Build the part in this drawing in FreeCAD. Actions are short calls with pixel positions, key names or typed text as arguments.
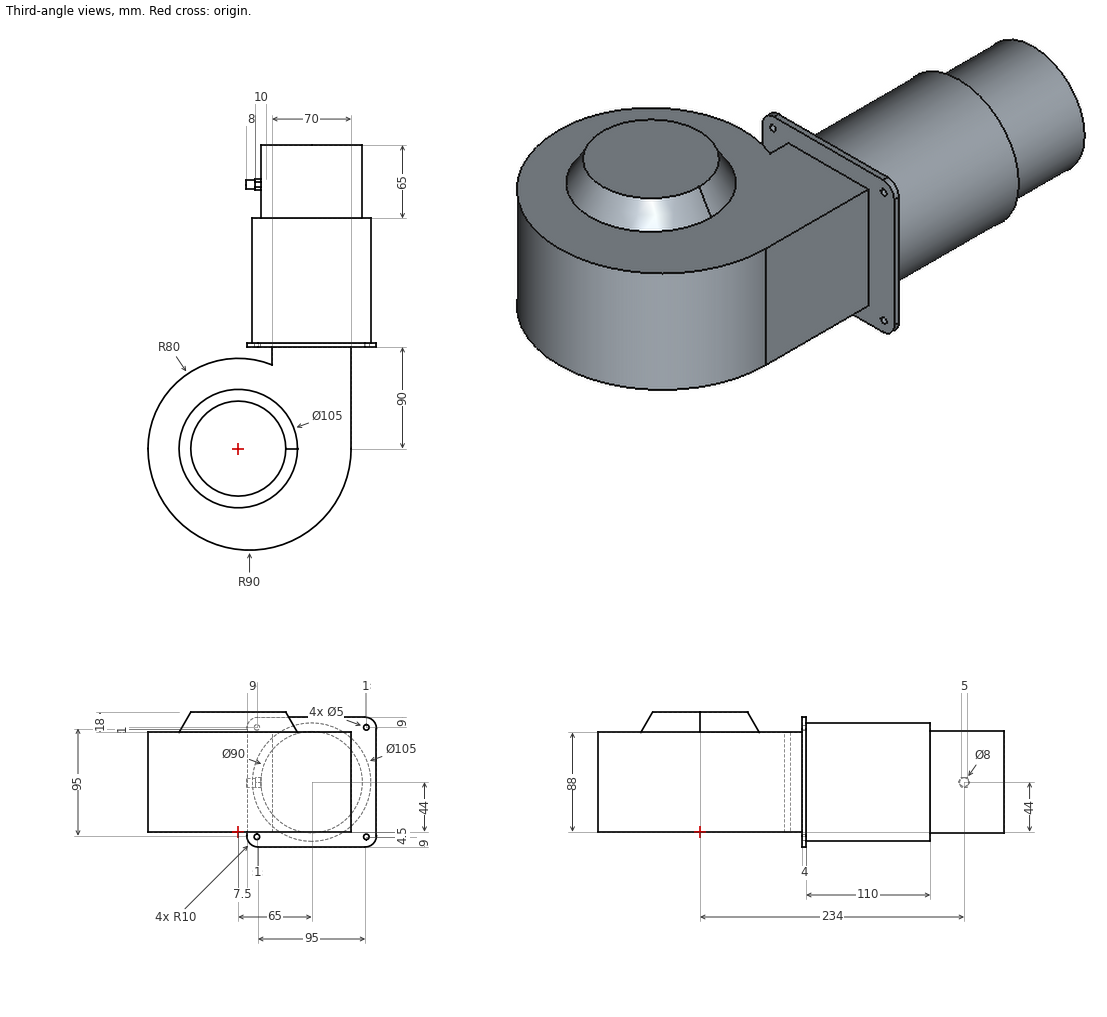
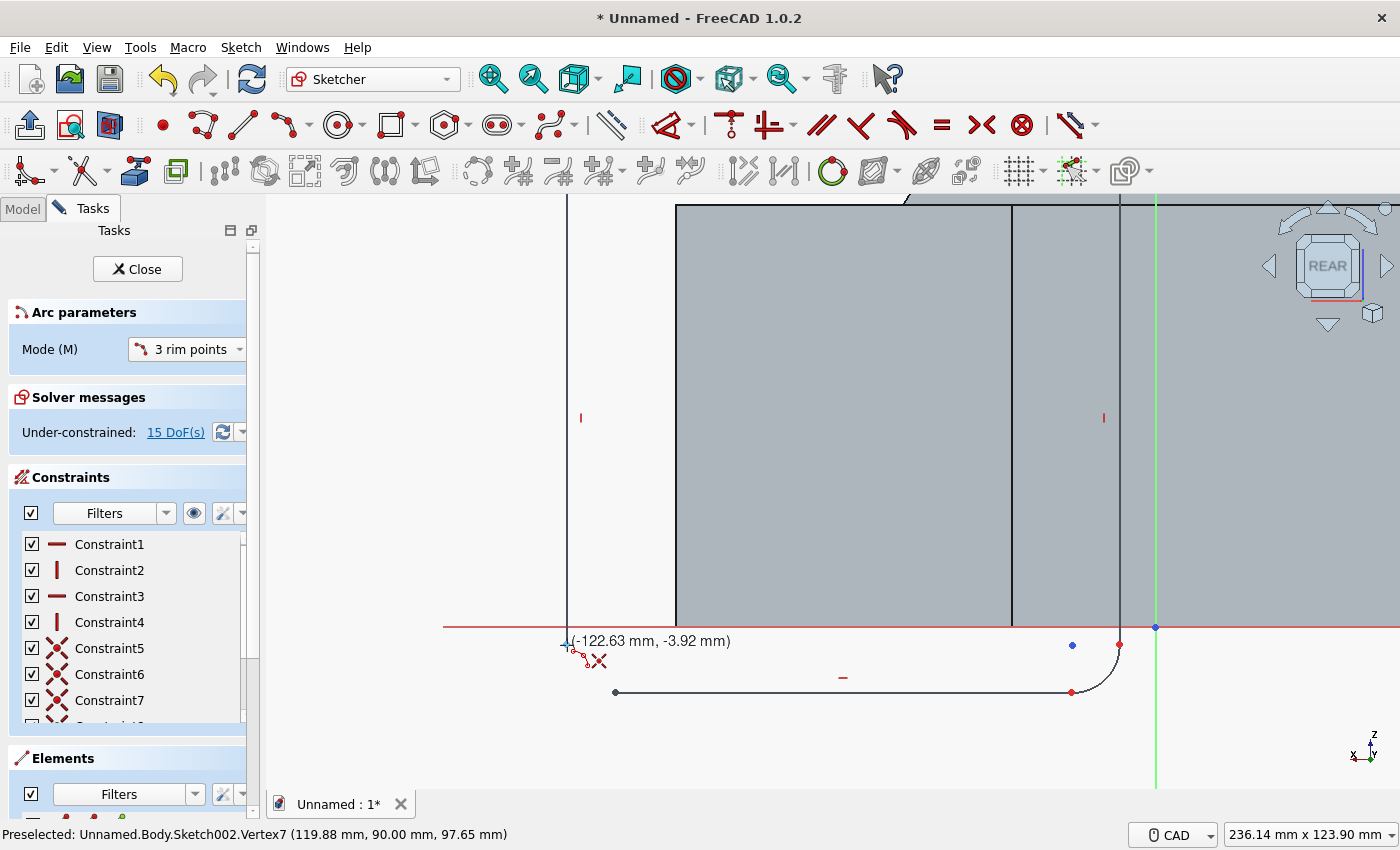
click(567, 645)
click(615, 693)
click(582, 678)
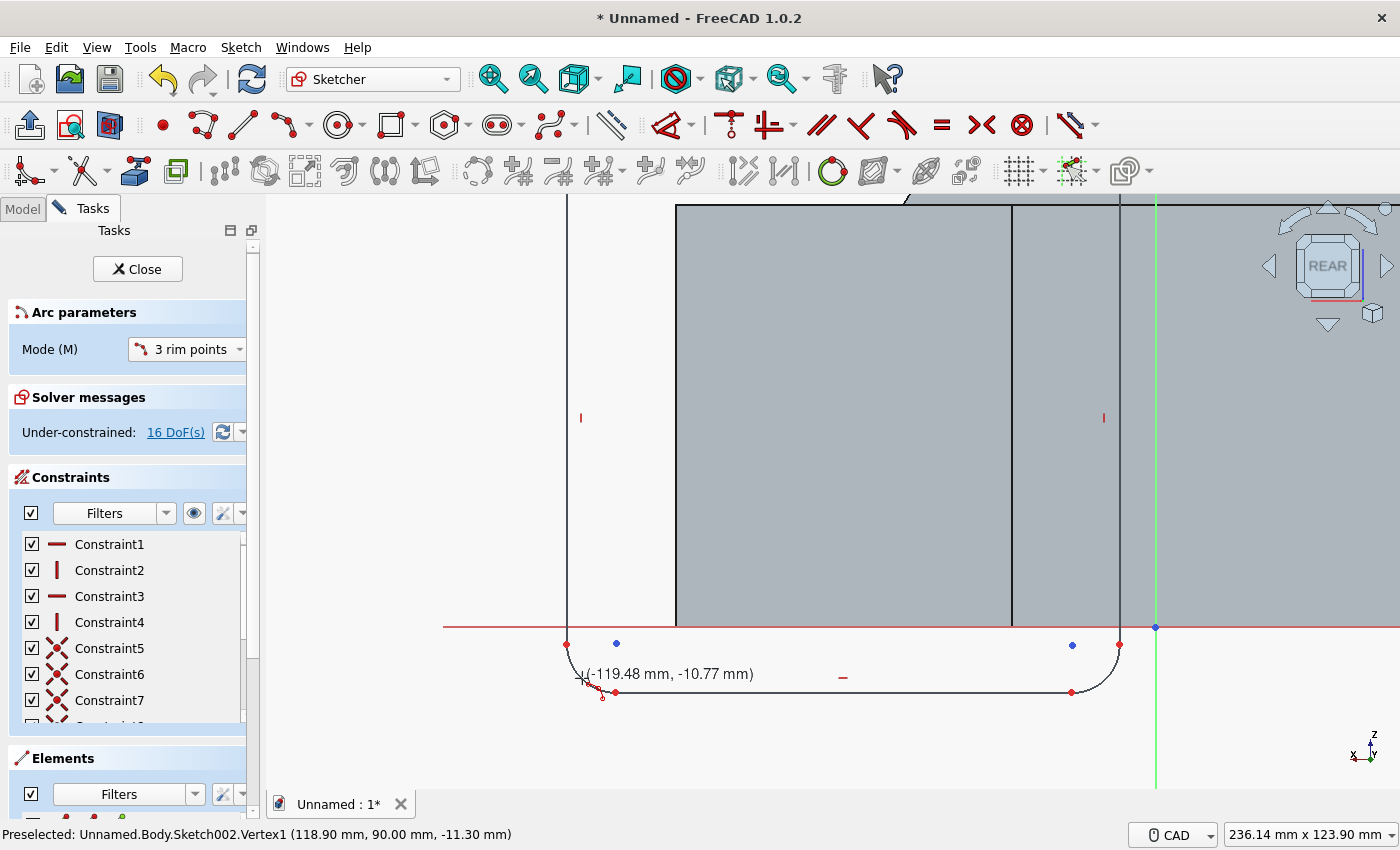
click(338, 126)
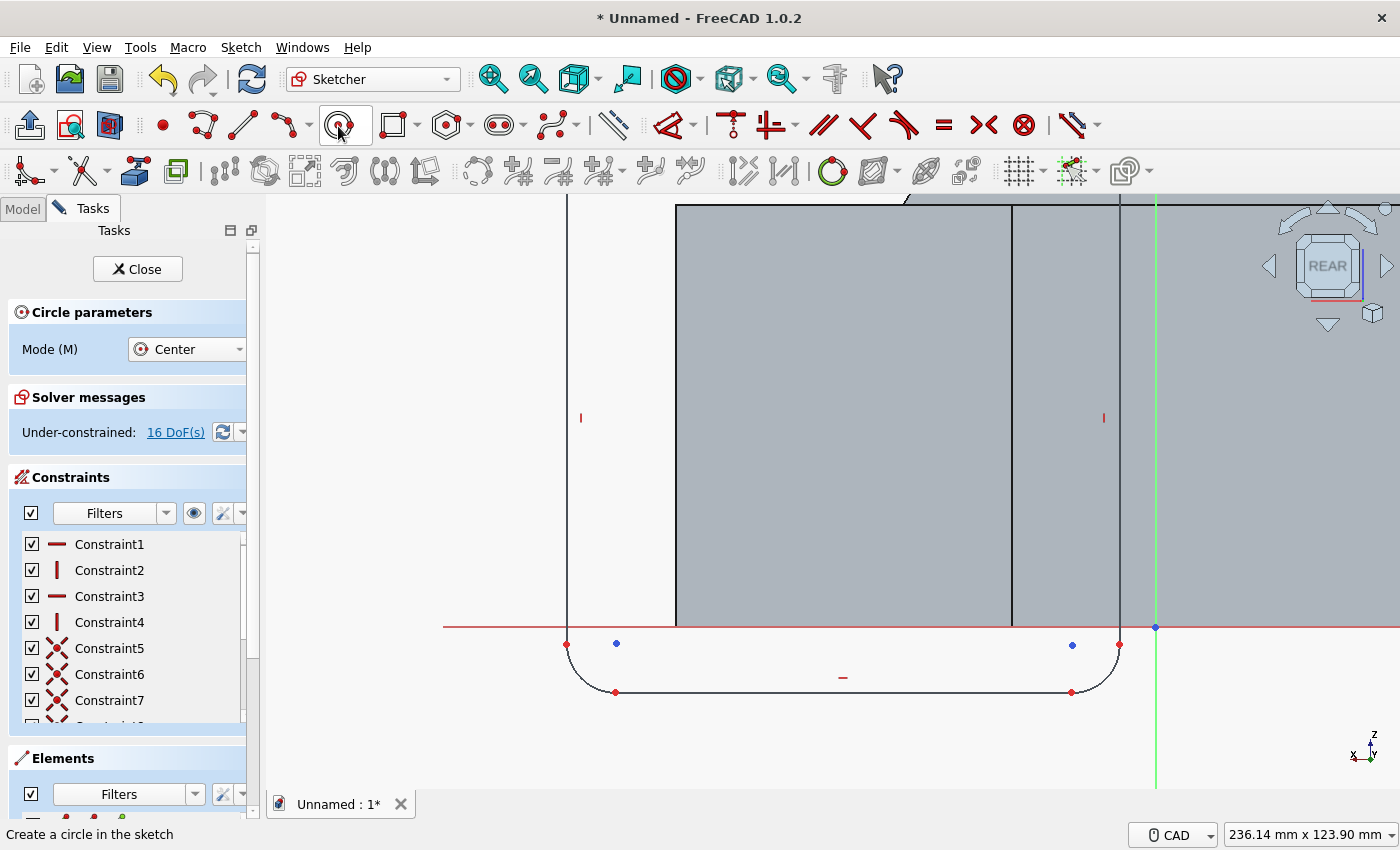
scroll(567, 645, down, 2)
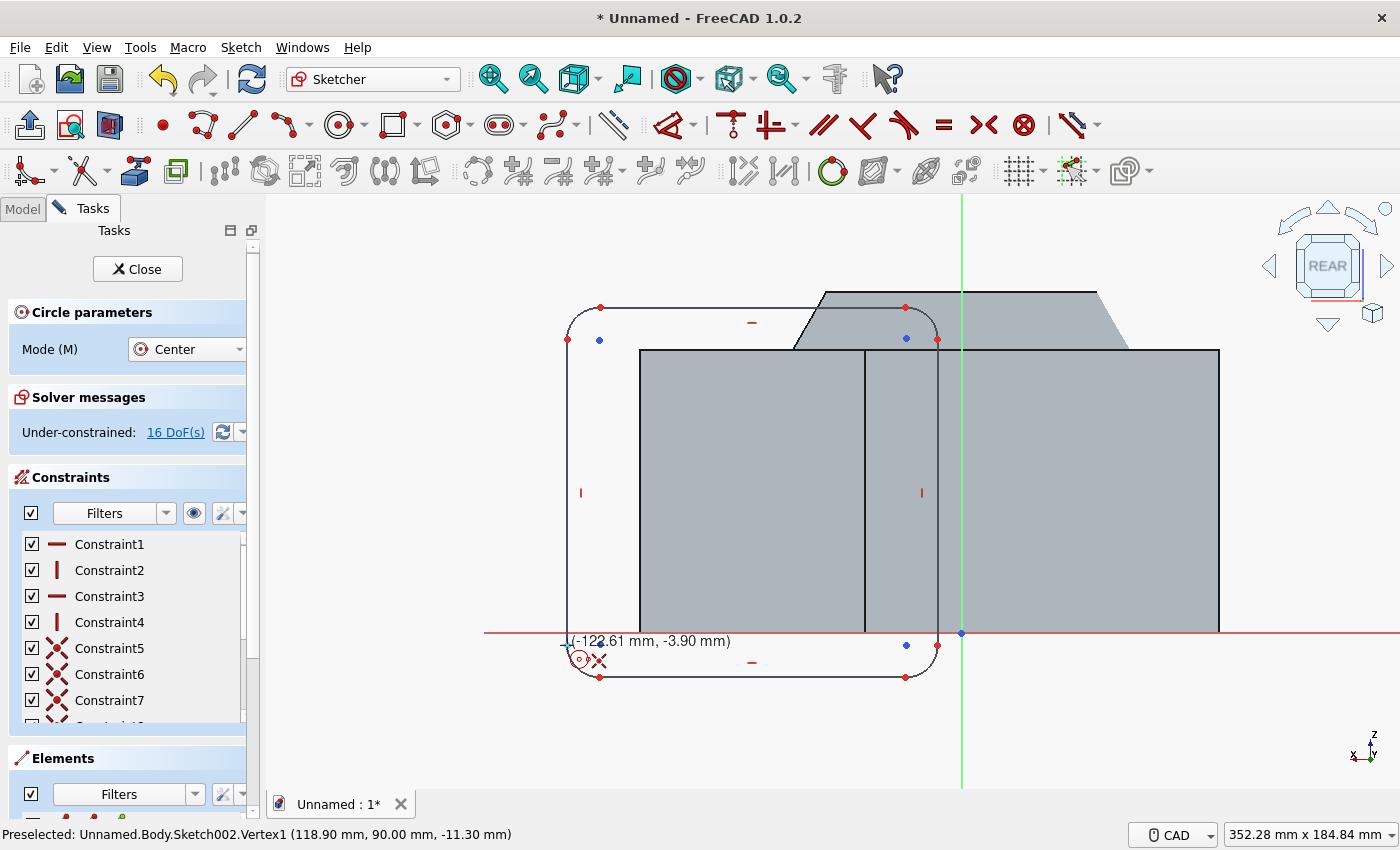
scroll(596, 336, up, 7)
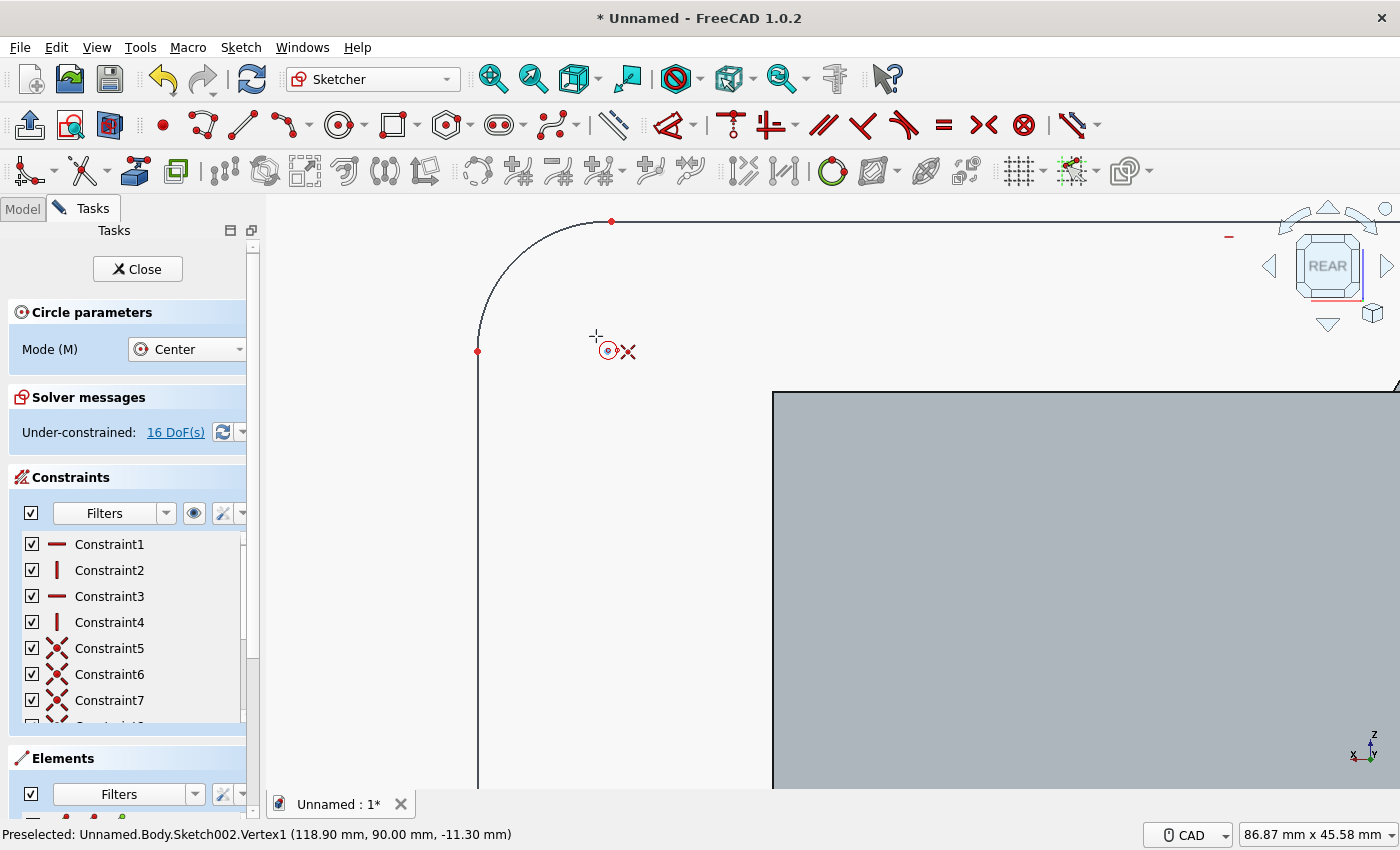
click(597, 334)
click(620, 311)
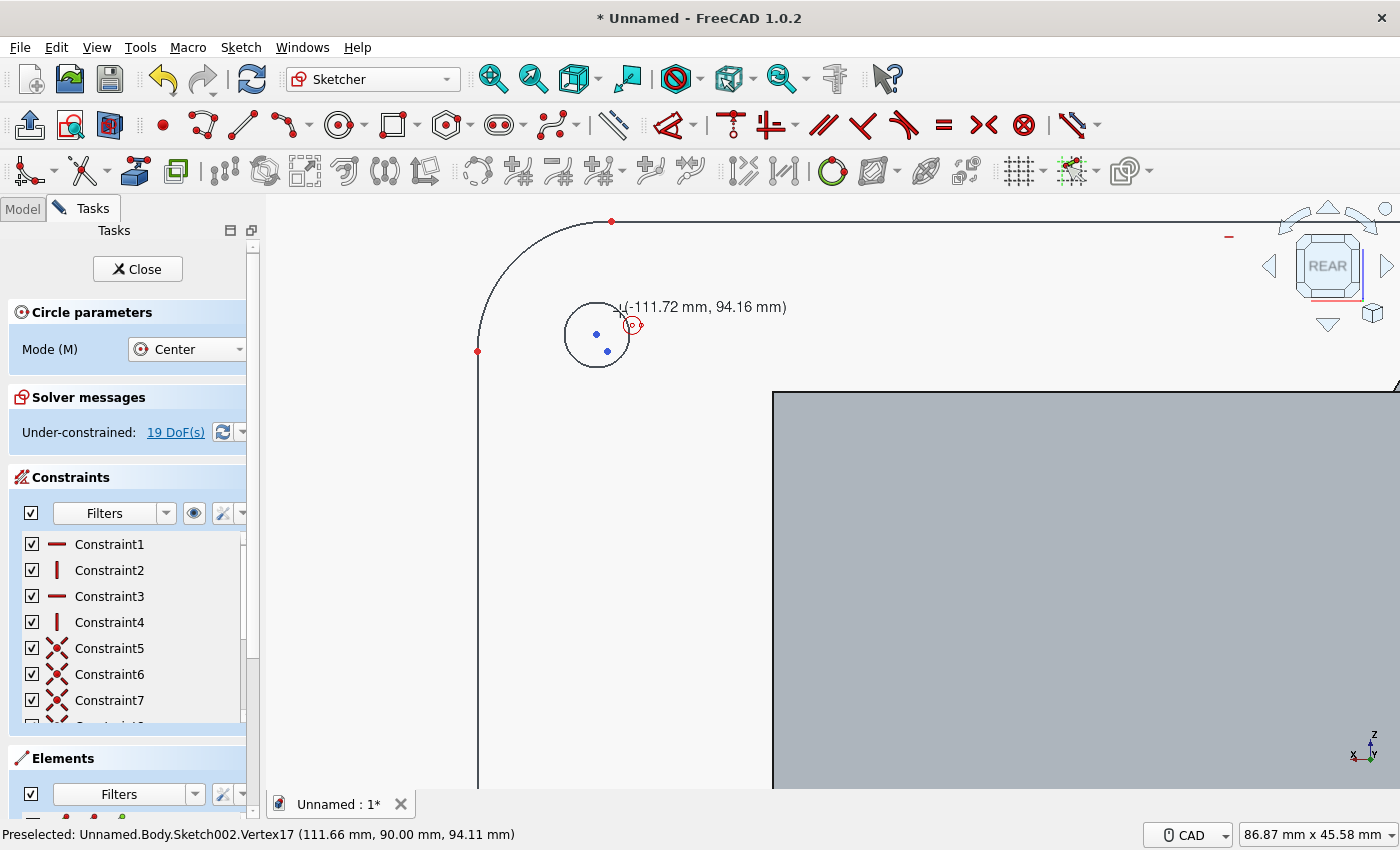
scroll(596, 336, down, 7)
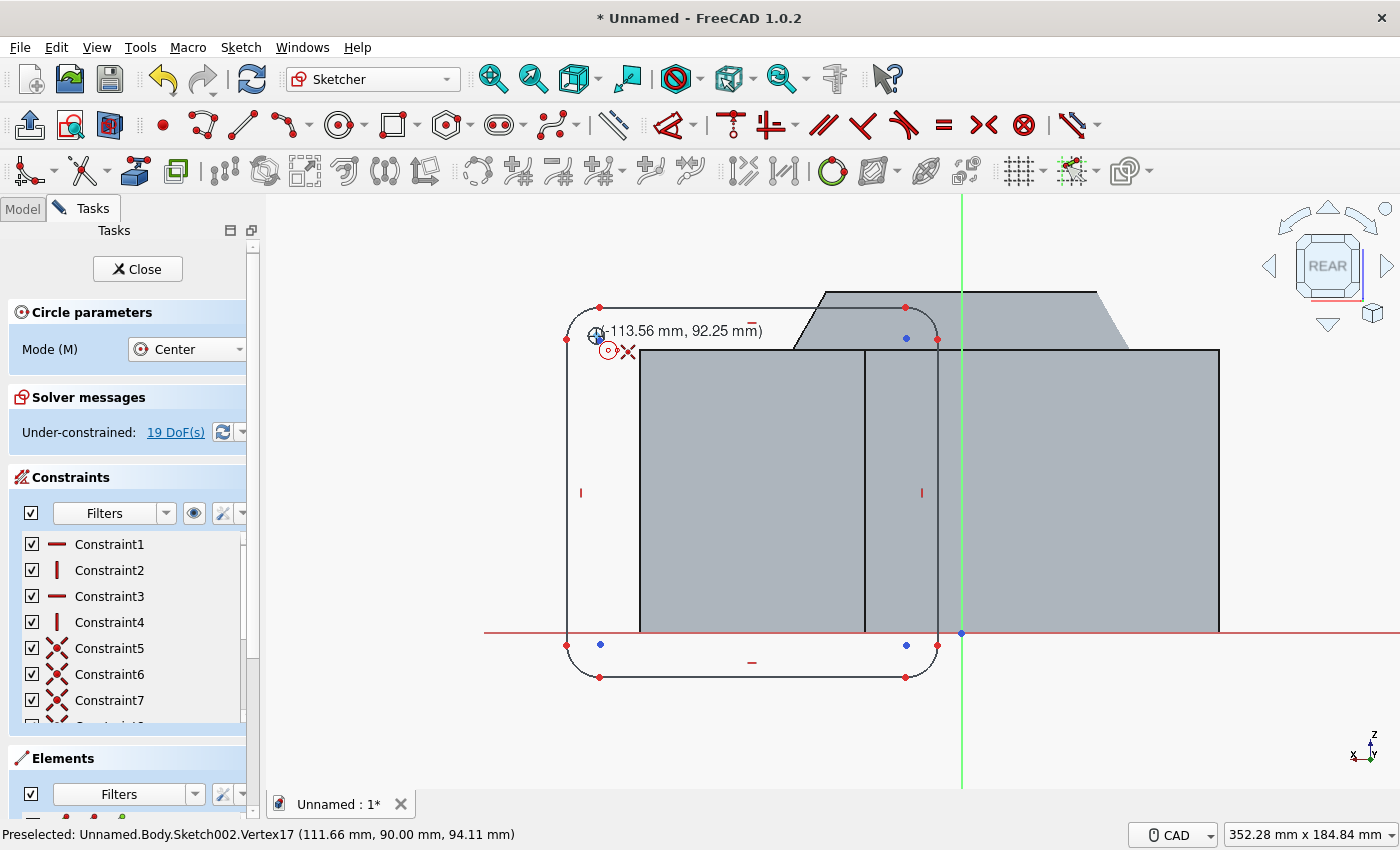
scroll(909, 336, up, 7)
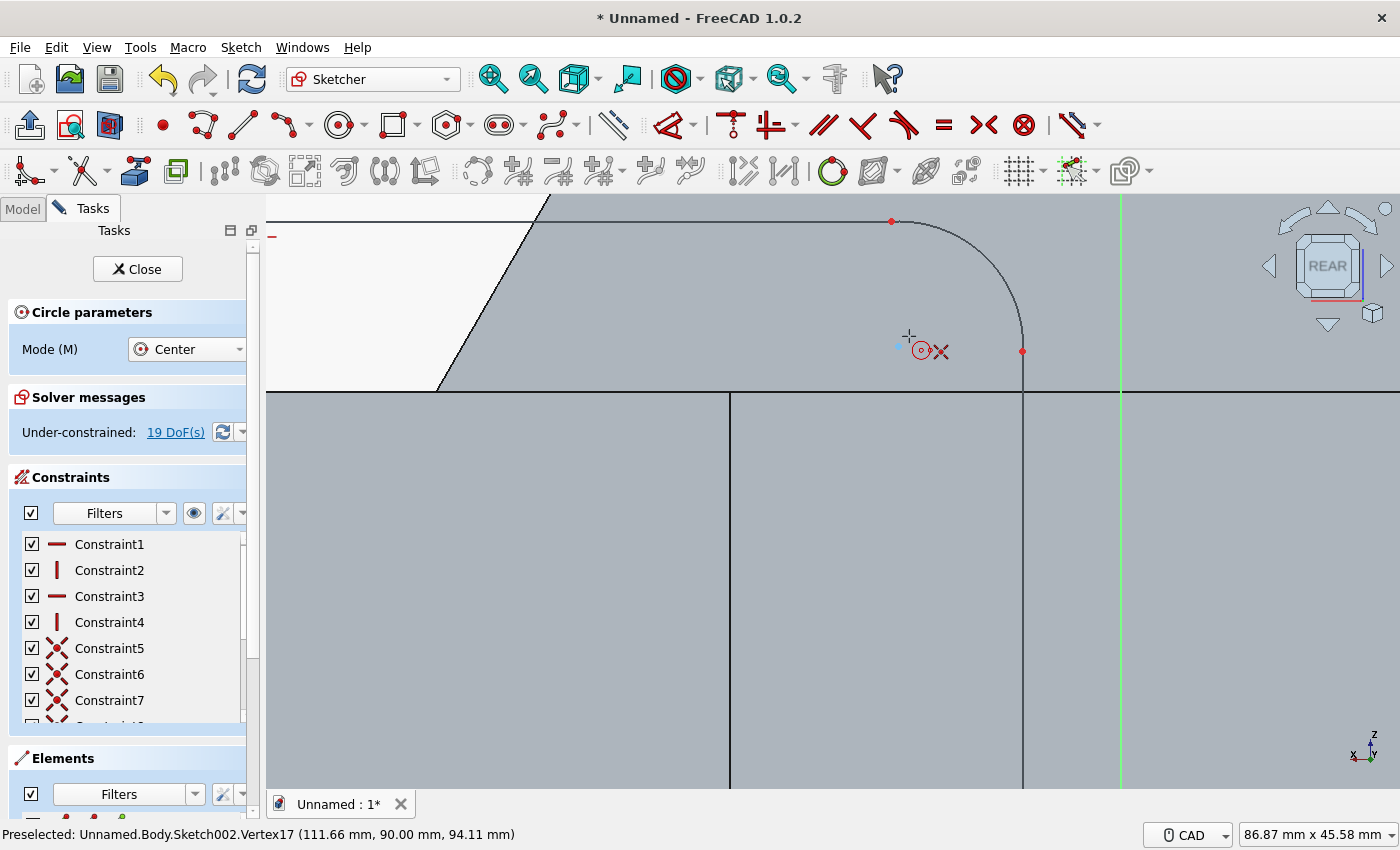
click(906, 334)
click(929, 311)